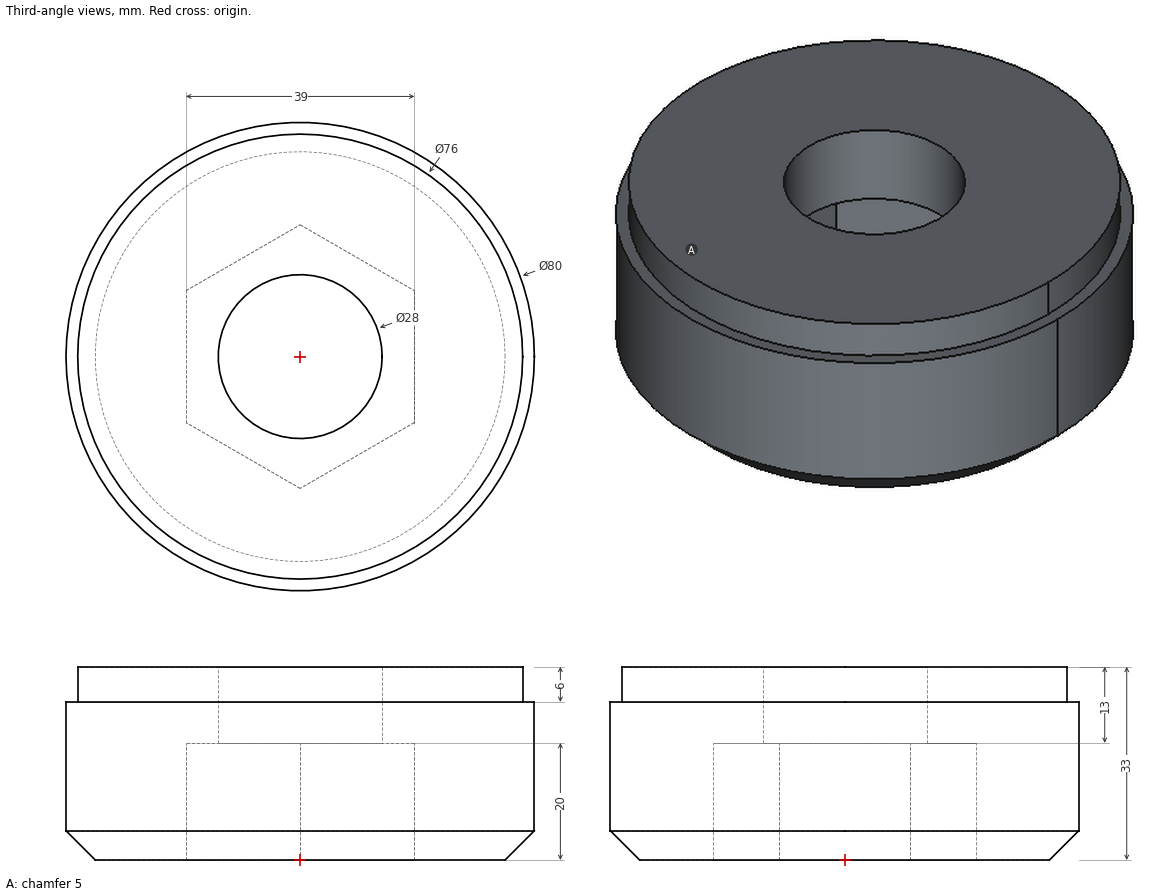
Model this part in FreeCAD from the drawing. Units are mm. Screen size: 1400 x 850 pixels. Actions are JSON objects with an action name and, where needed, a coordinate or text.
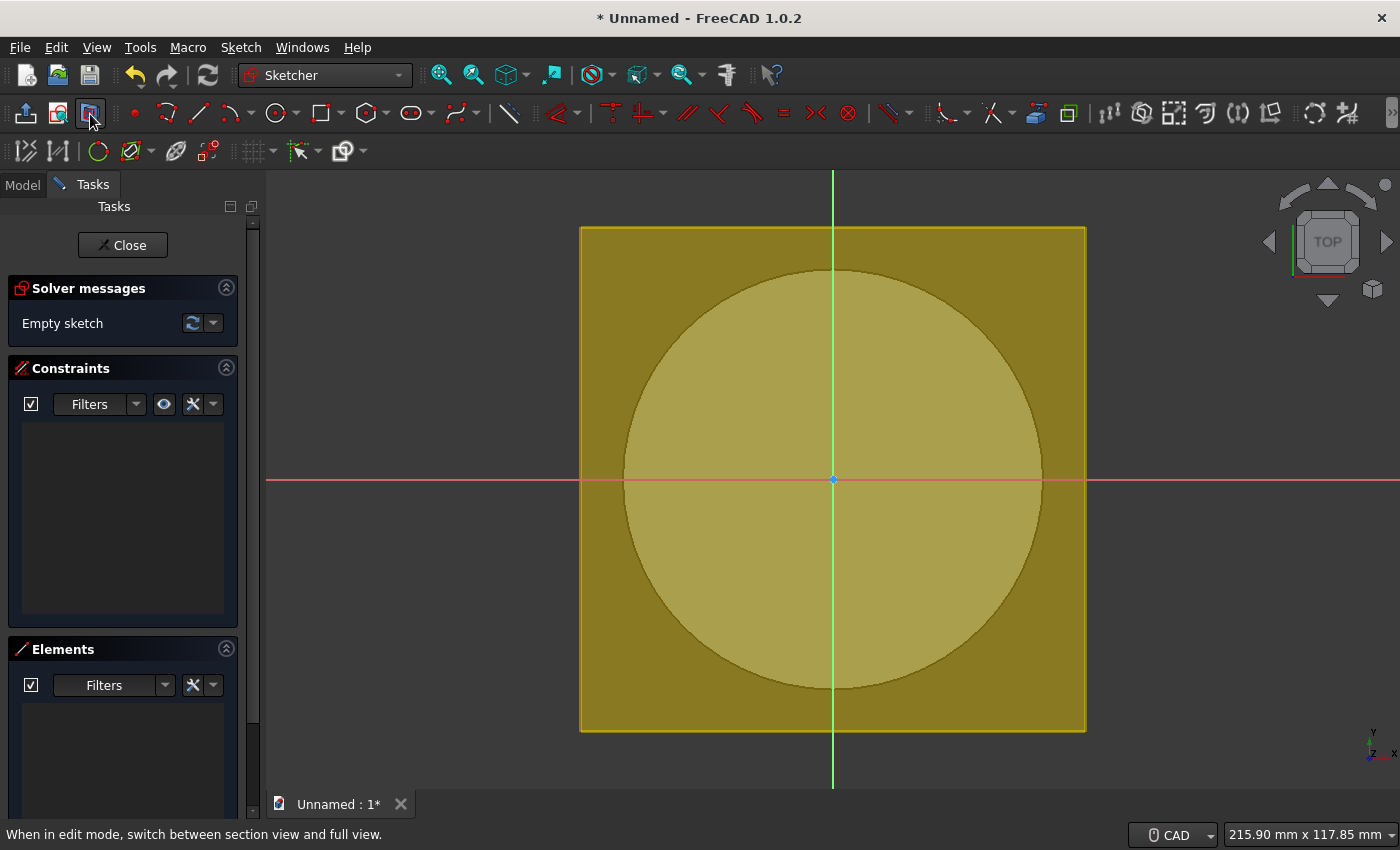
{"action": "left_click", "coordinate": [276, 114]}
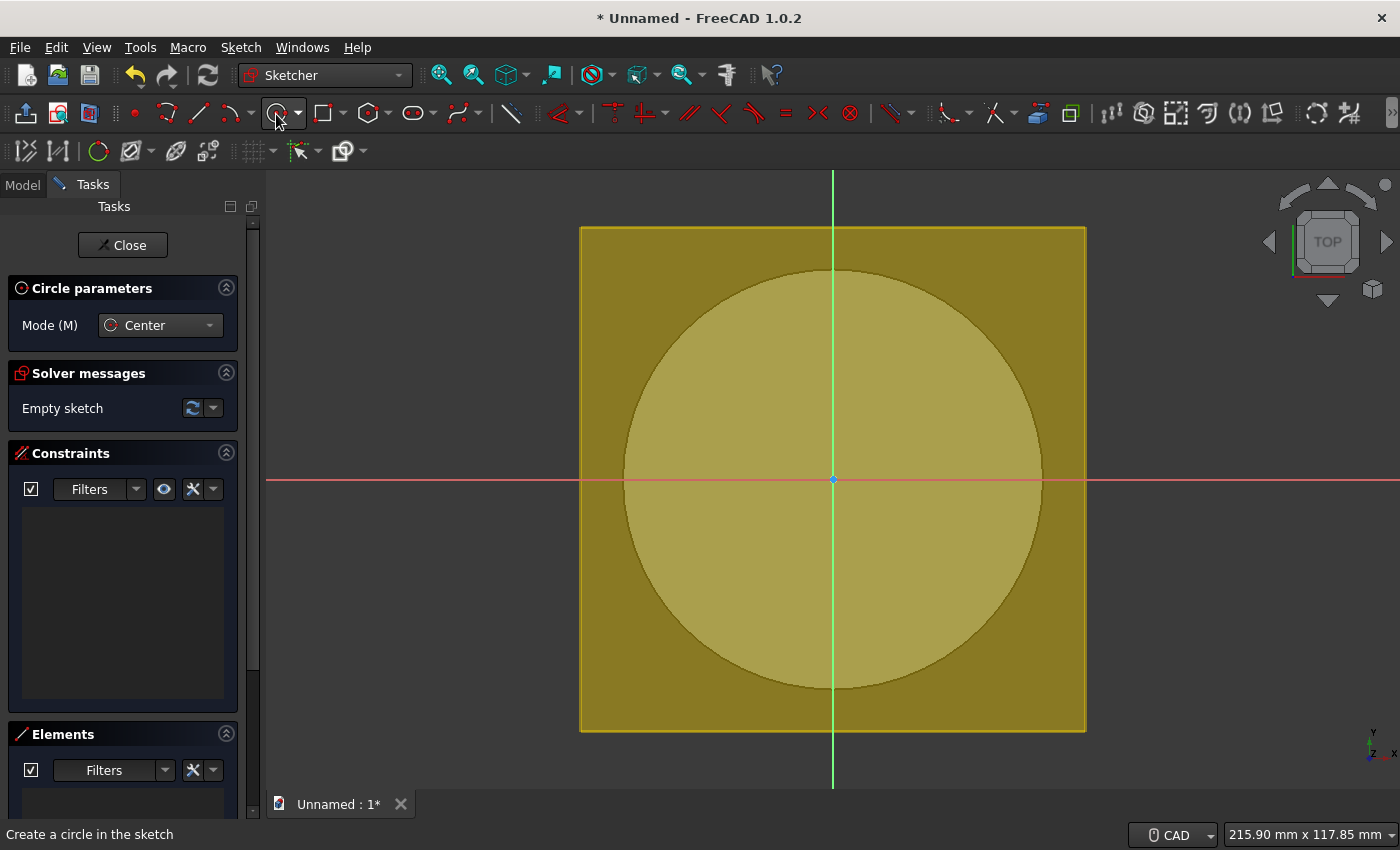
{"action": "left_click", "coordinate": [833, 480]}
{"action": "left_click", "coordinate": [982, 331]}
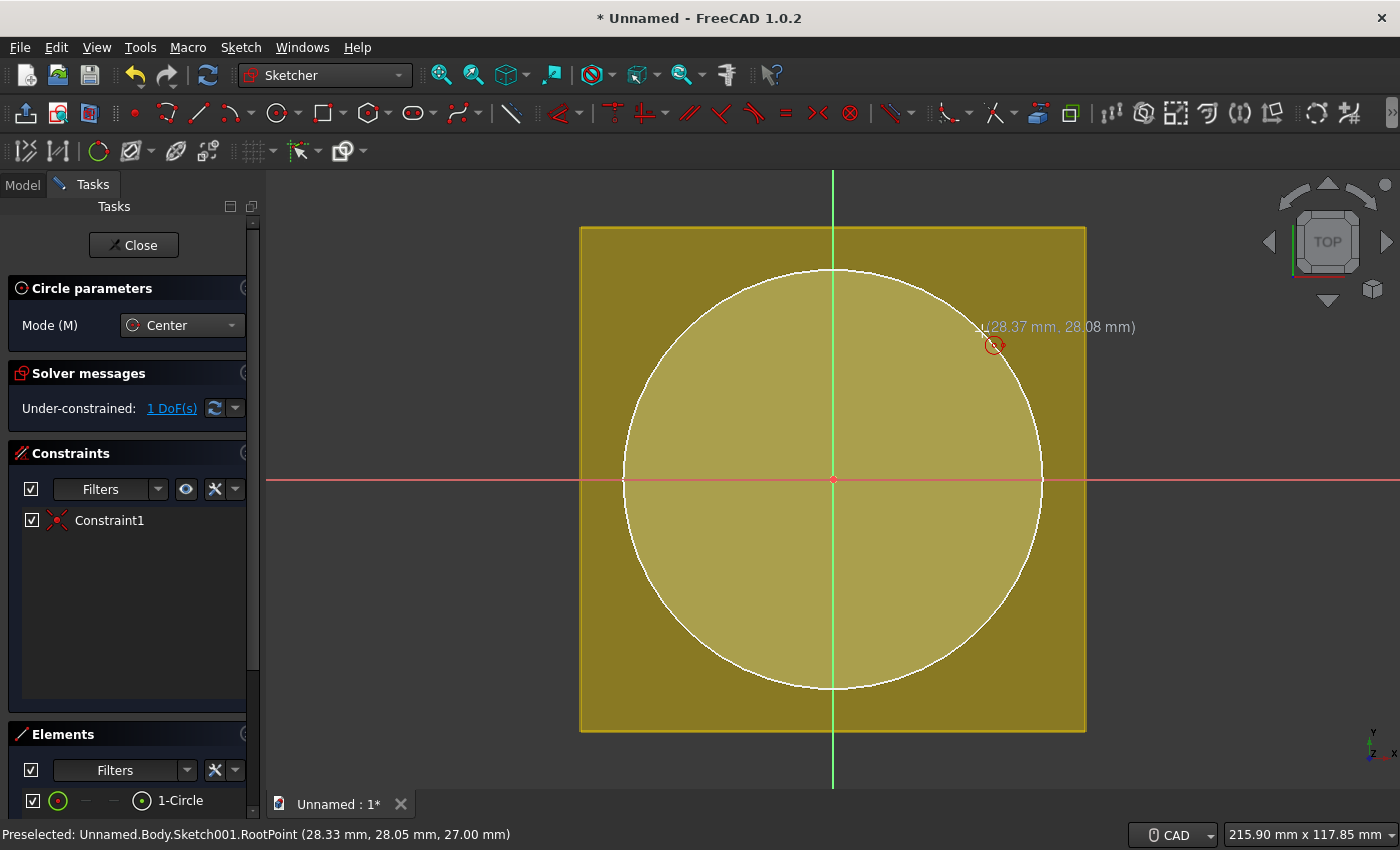
{"action": "left_click", "coordinate": [833, 480]}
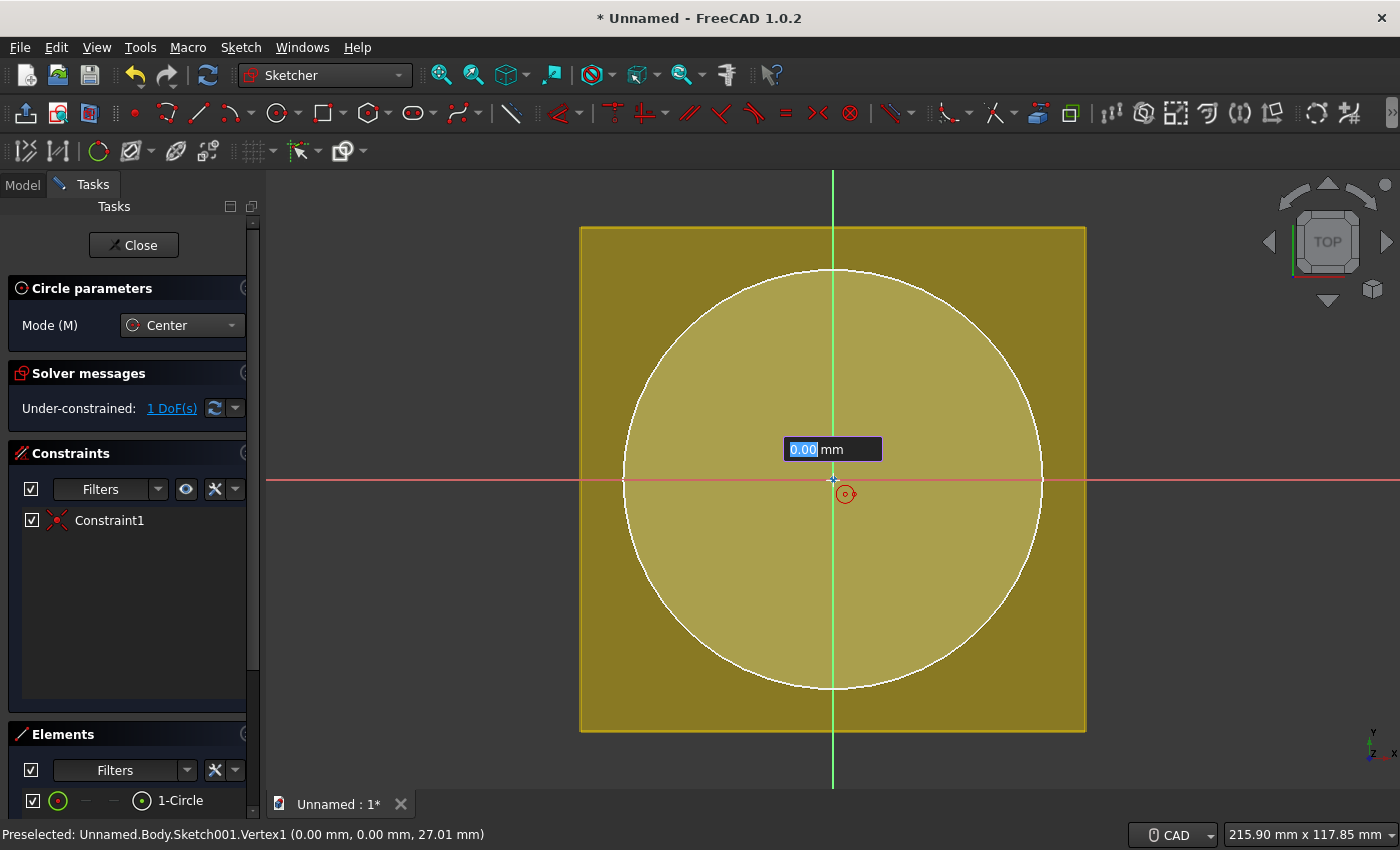
{"action": "scroll", "coordinate": [974, 338], "scroll_direction": "up", "scroll_amount": 3}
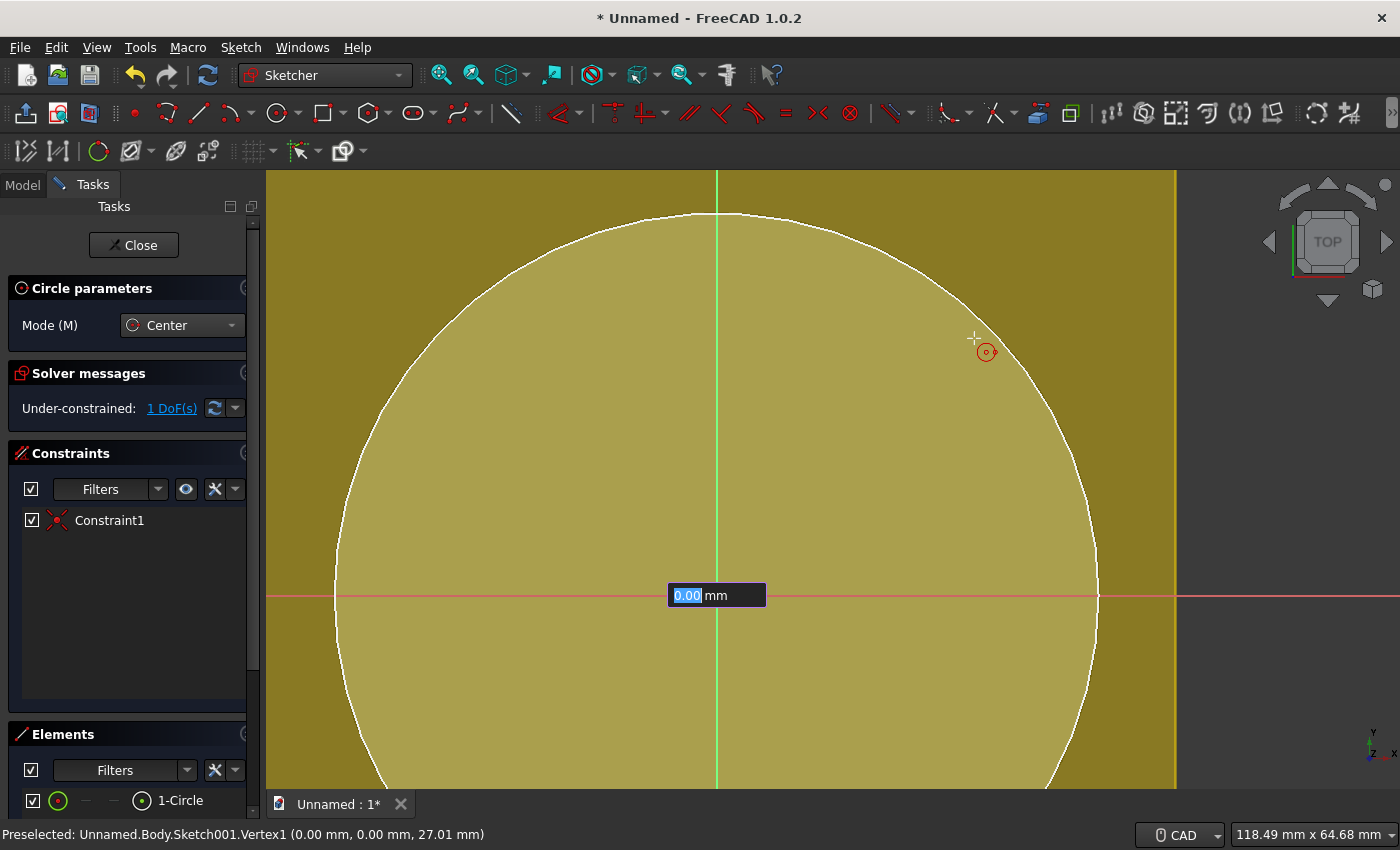
{"action": "left_click", "coordinate": [974, 338]}
{"action": "key", "text": "Escape"}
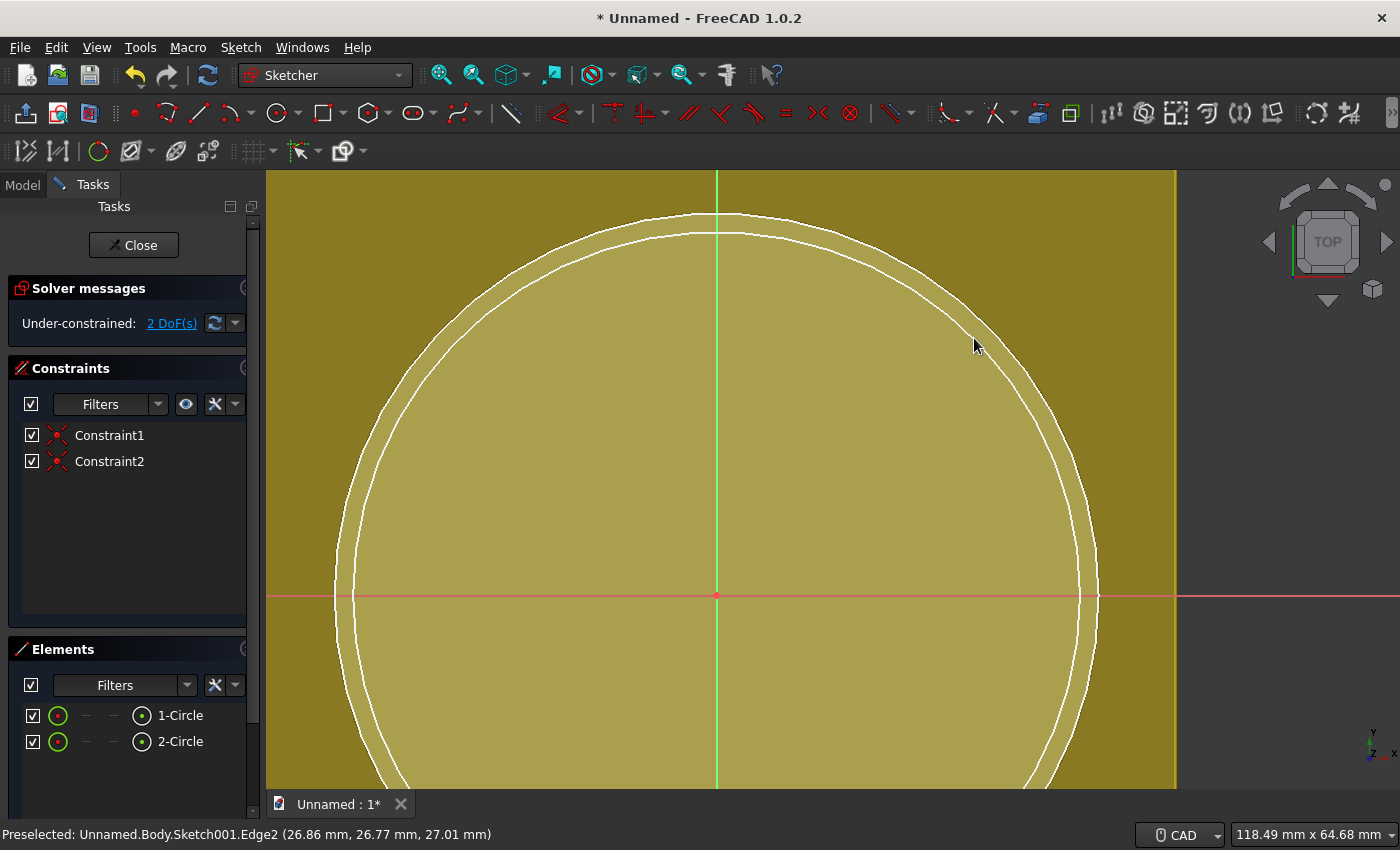
{"action": "left_click", "coordinate": [558, 114]}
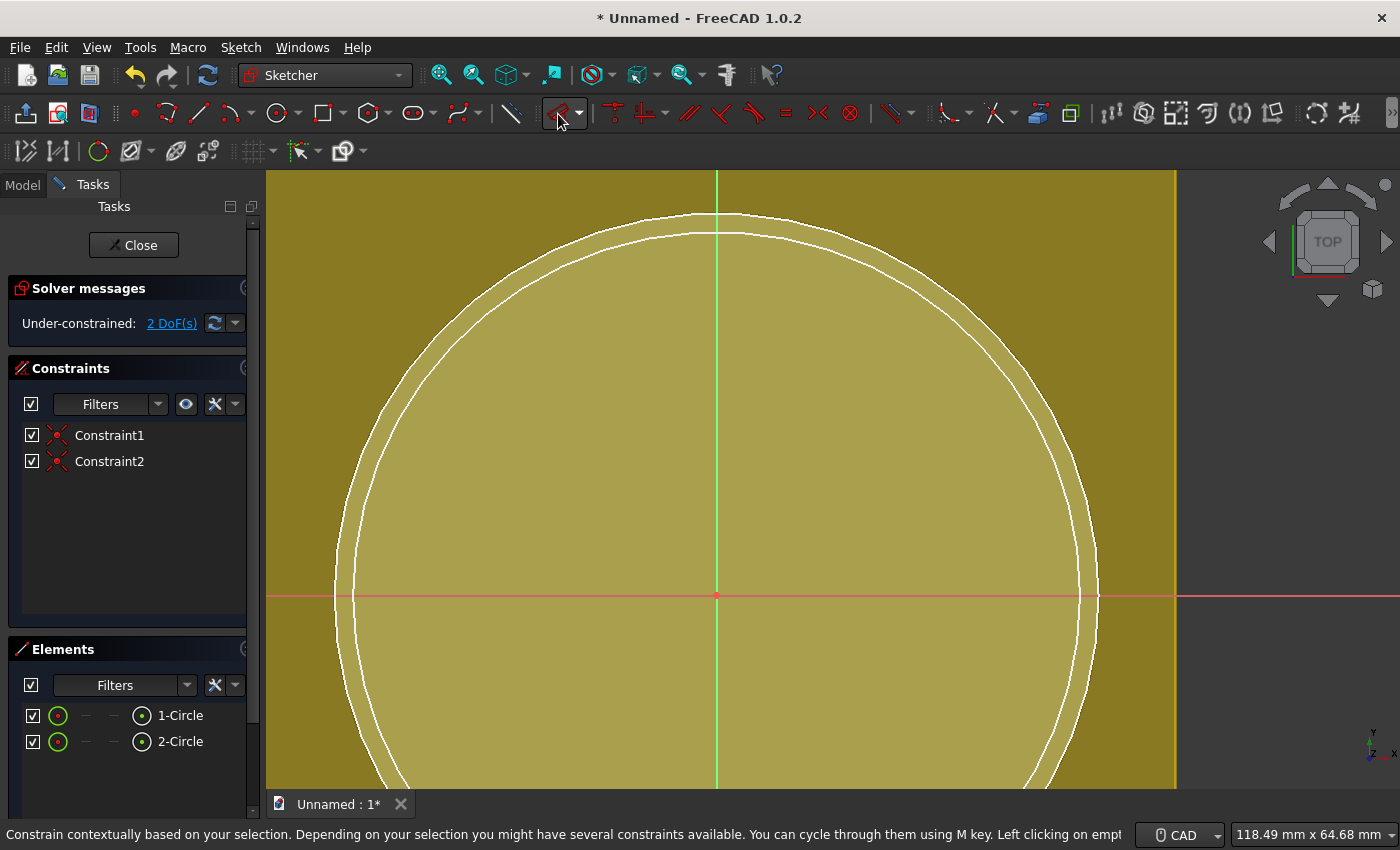
{"action": "left_click", "coordinate": [986, 325]}
{"action": "left_click", "coordinate": [1009, 302]}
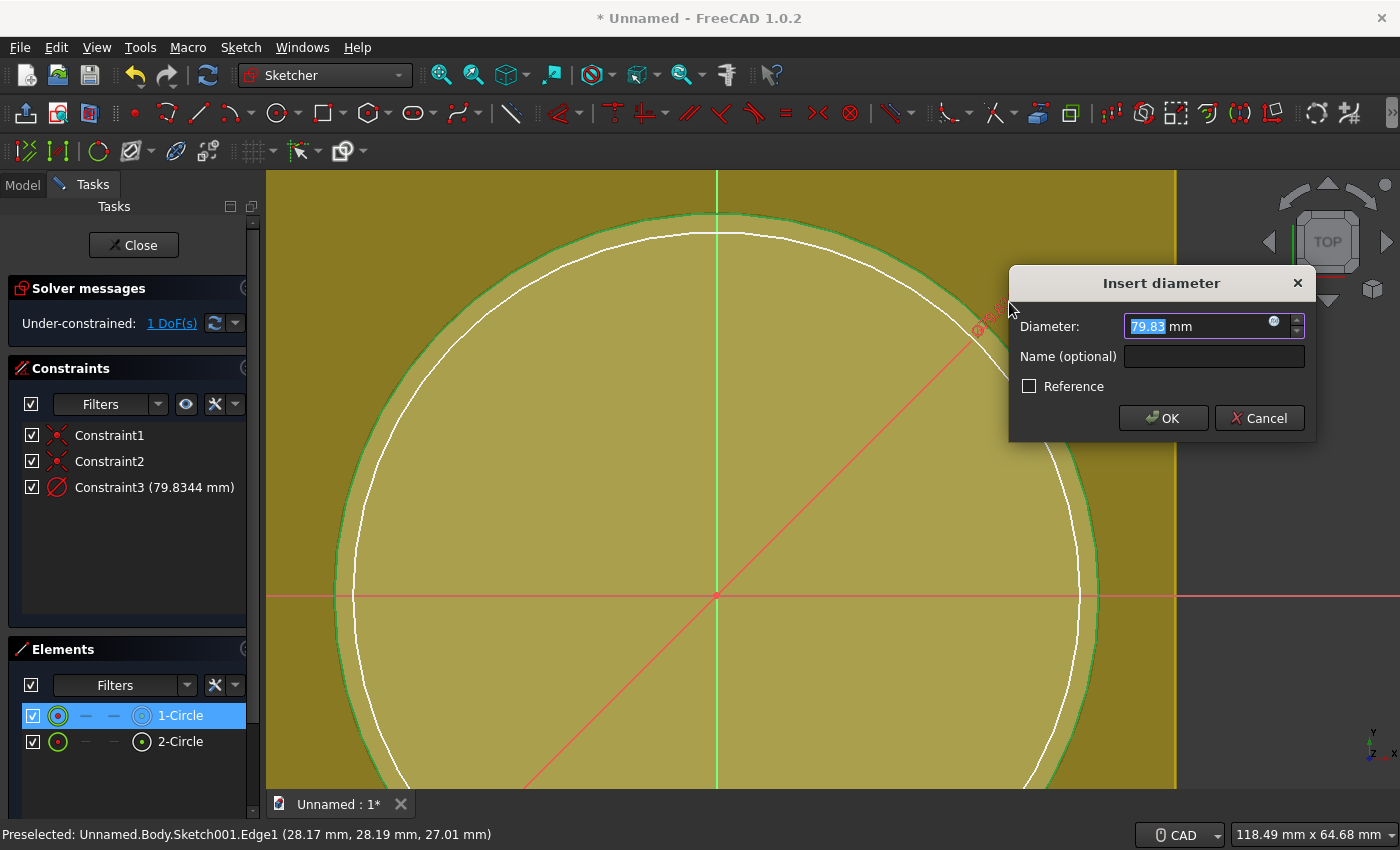
{"action": "type", "text": "80"}
{"action": "key", "text": "Return"}